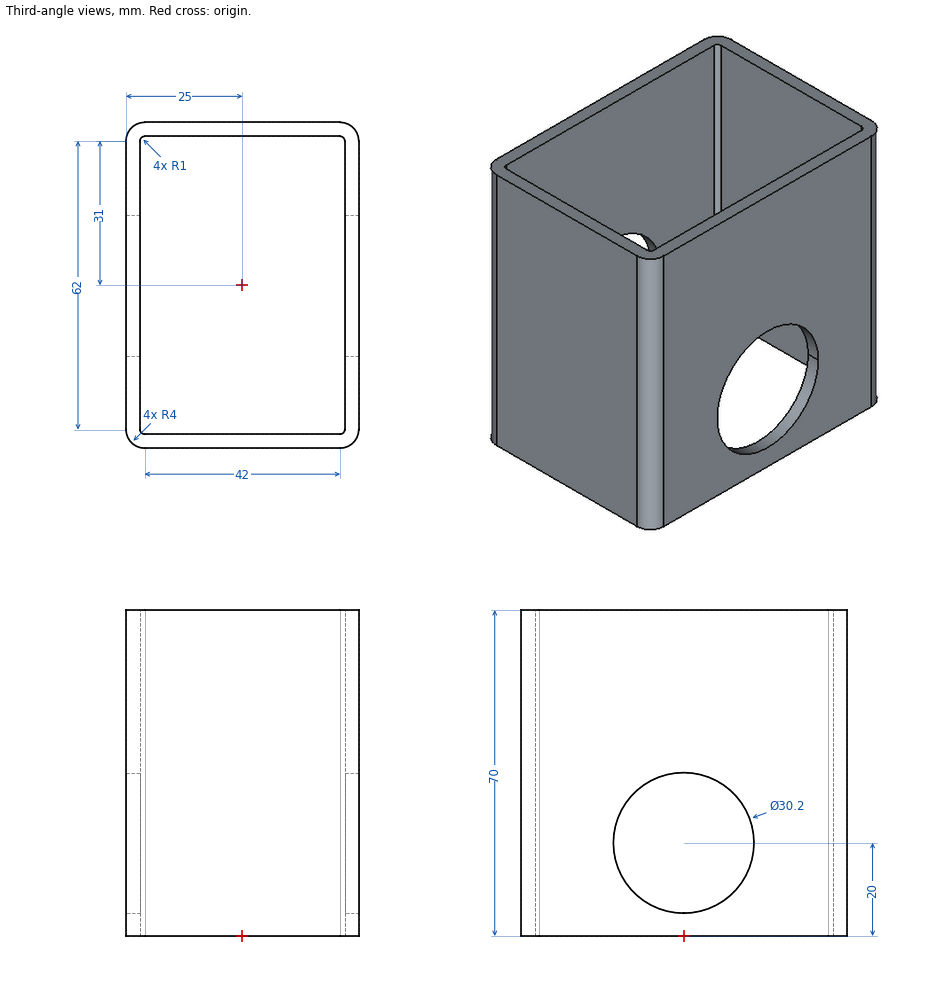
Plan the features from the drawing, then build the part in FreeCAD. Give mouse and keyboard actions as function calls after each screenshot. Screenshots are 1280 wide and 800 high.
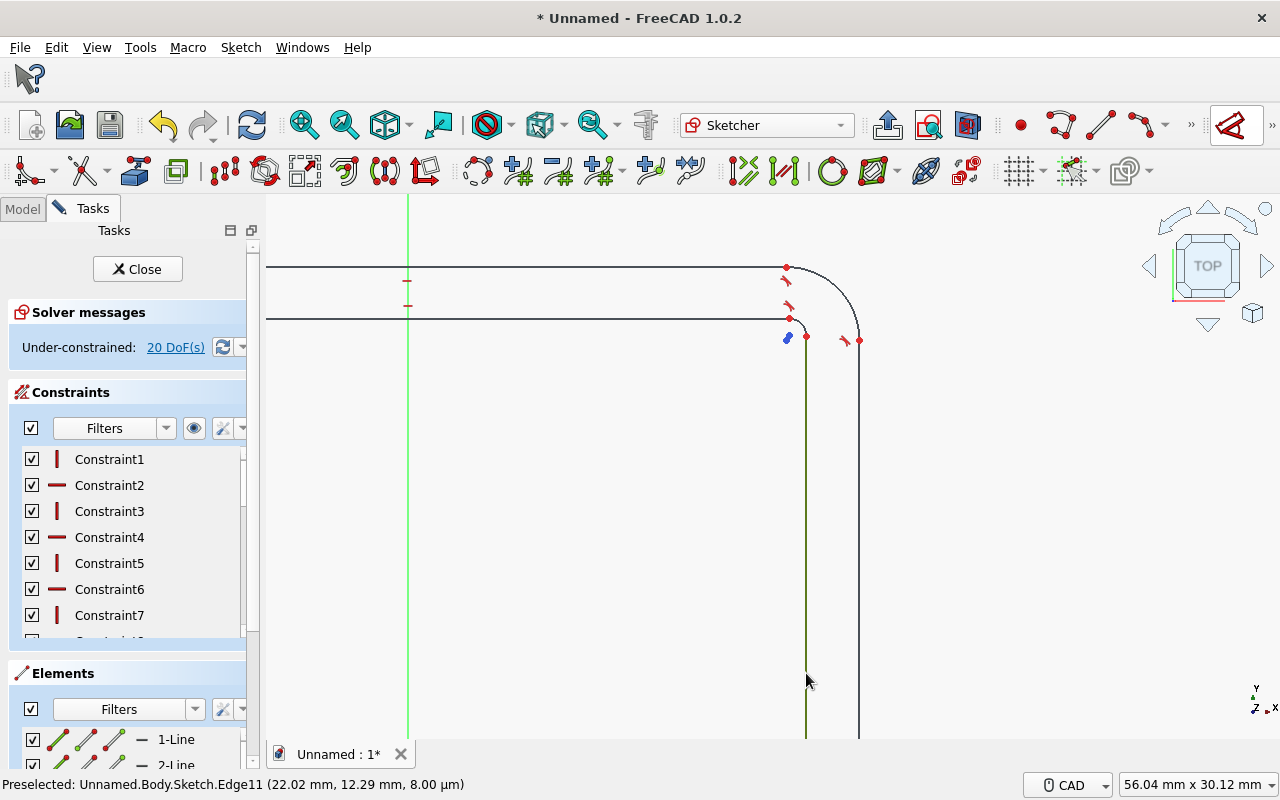
click(802, 324)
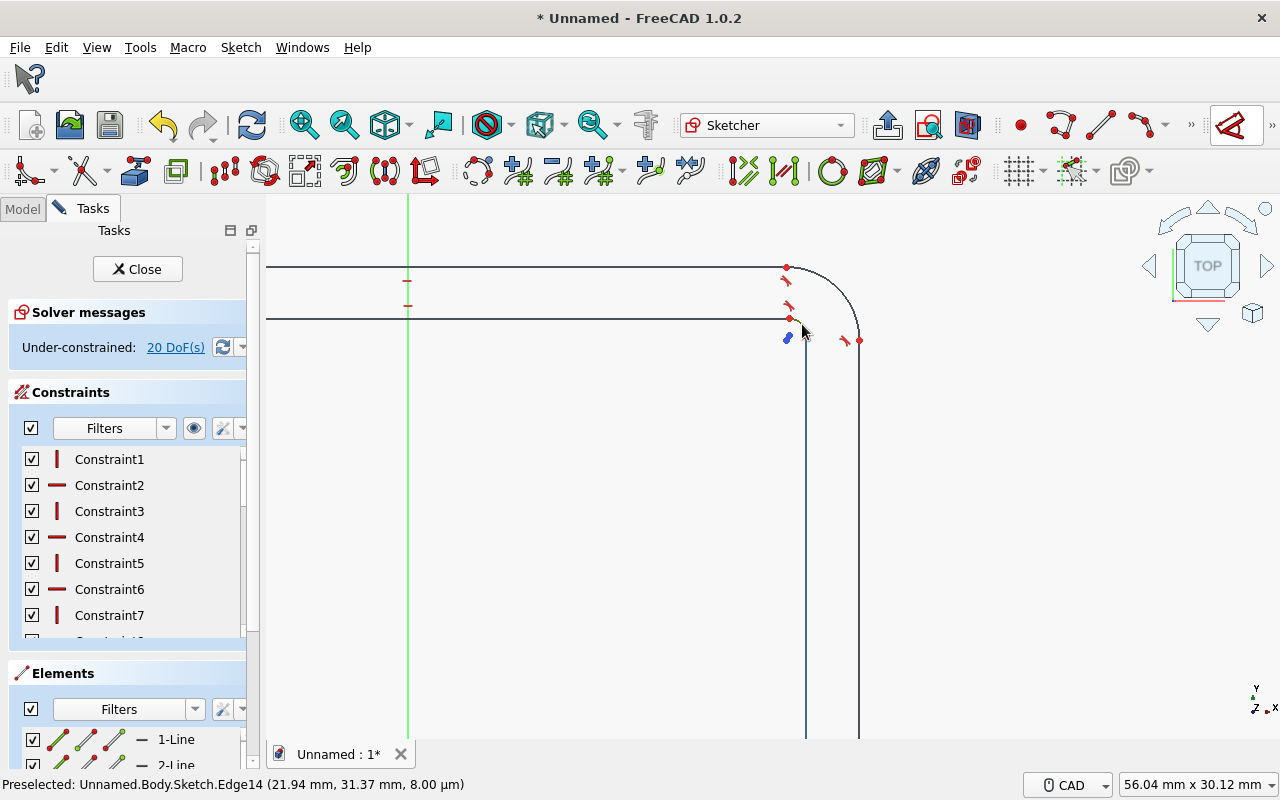
key(t)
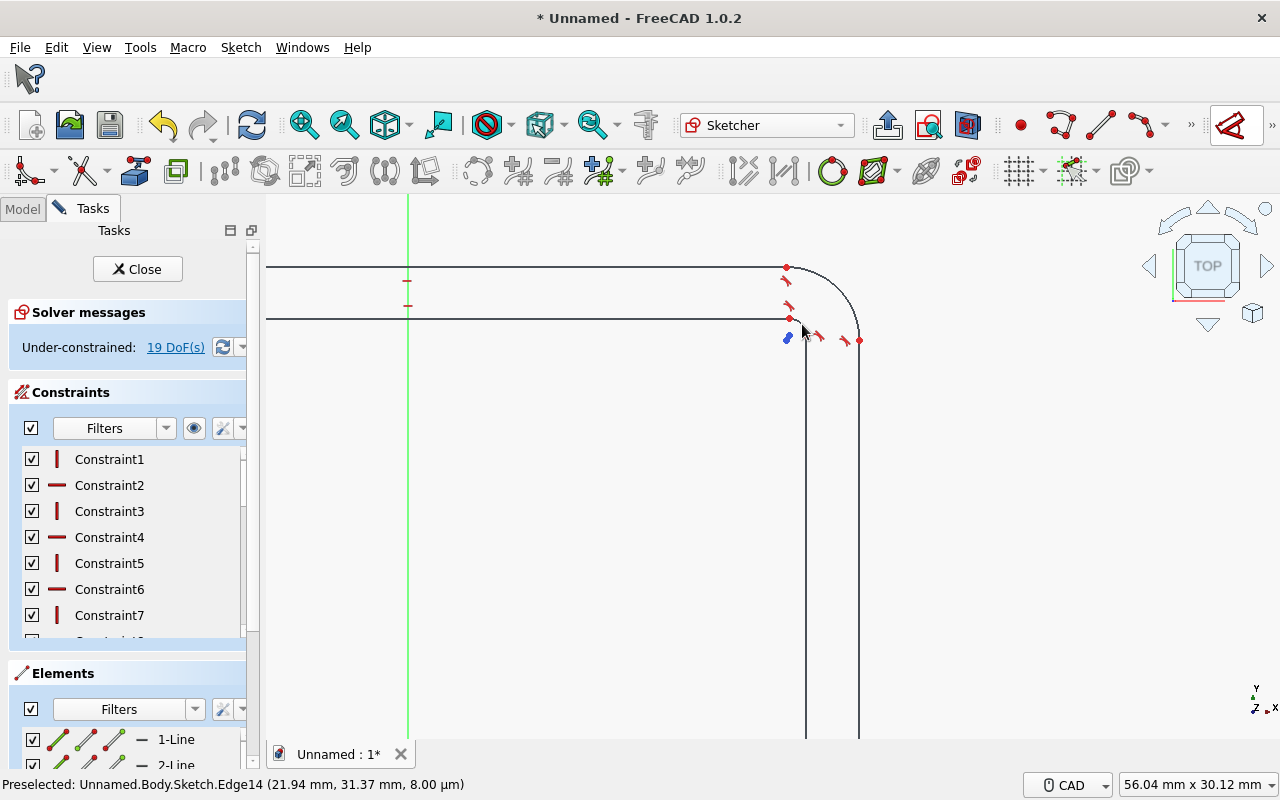
click(806, 672)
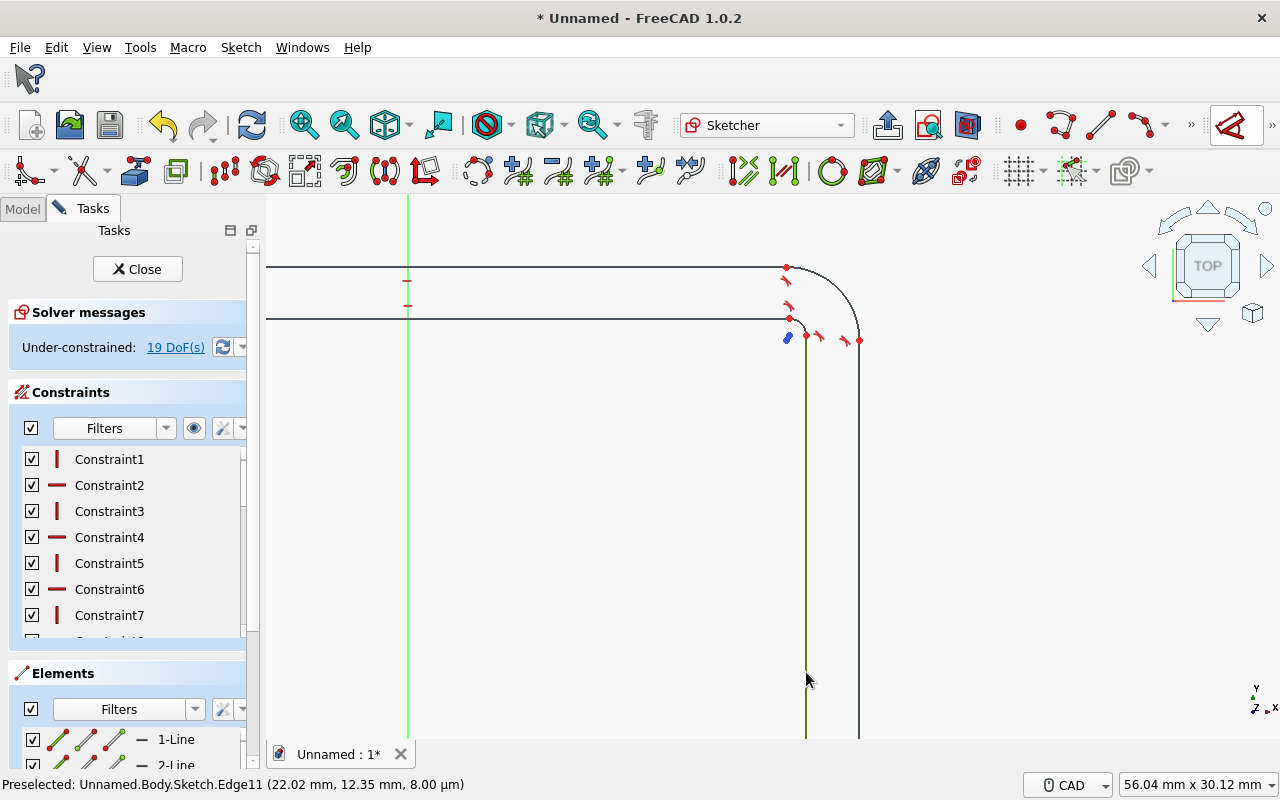
scroll(802, 326, down, 7)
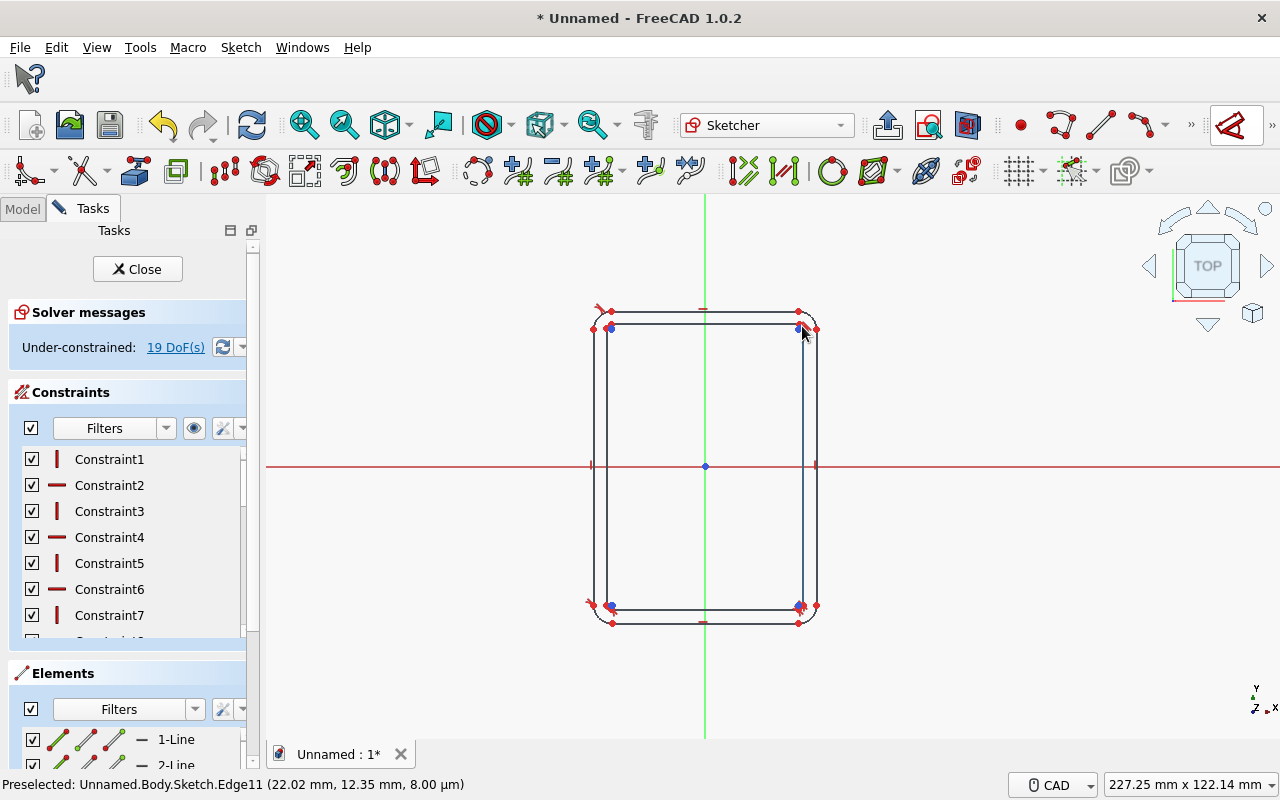
scroll(802, 609, up, 7)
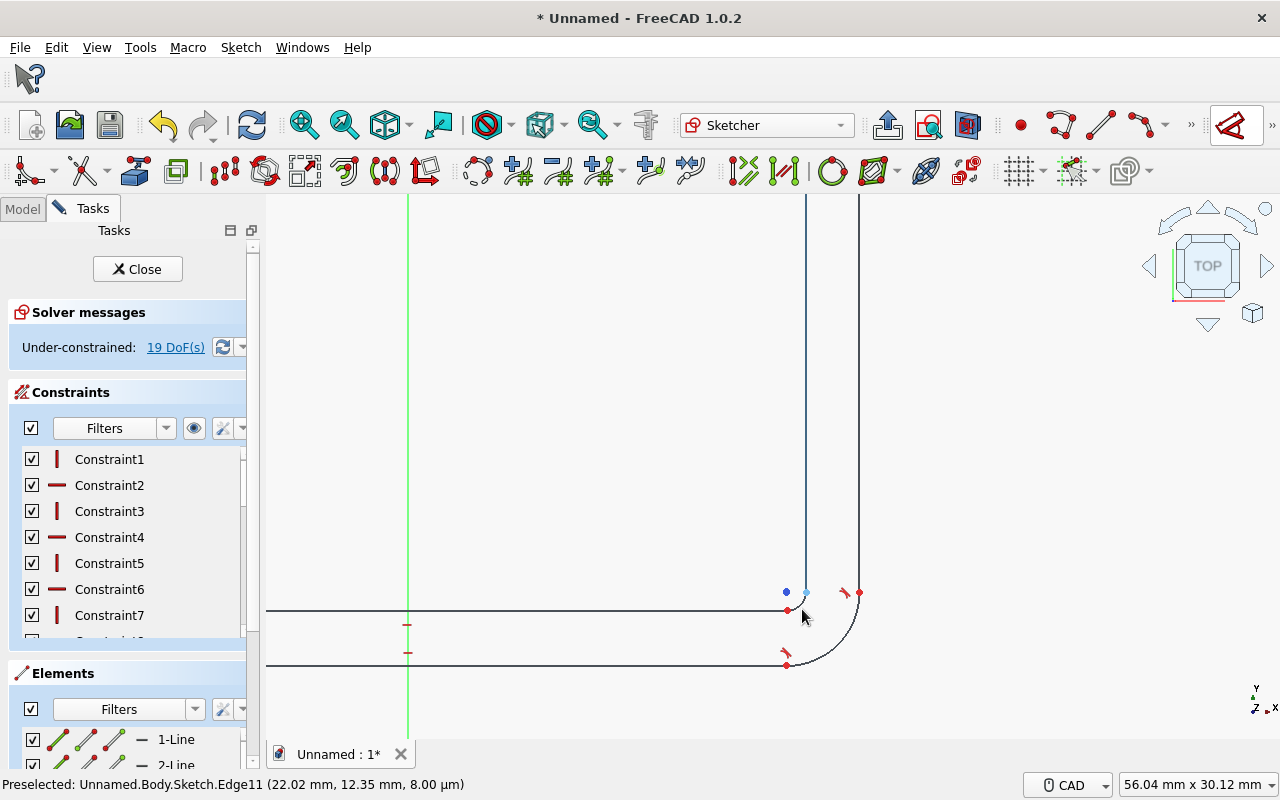
click(801, 605)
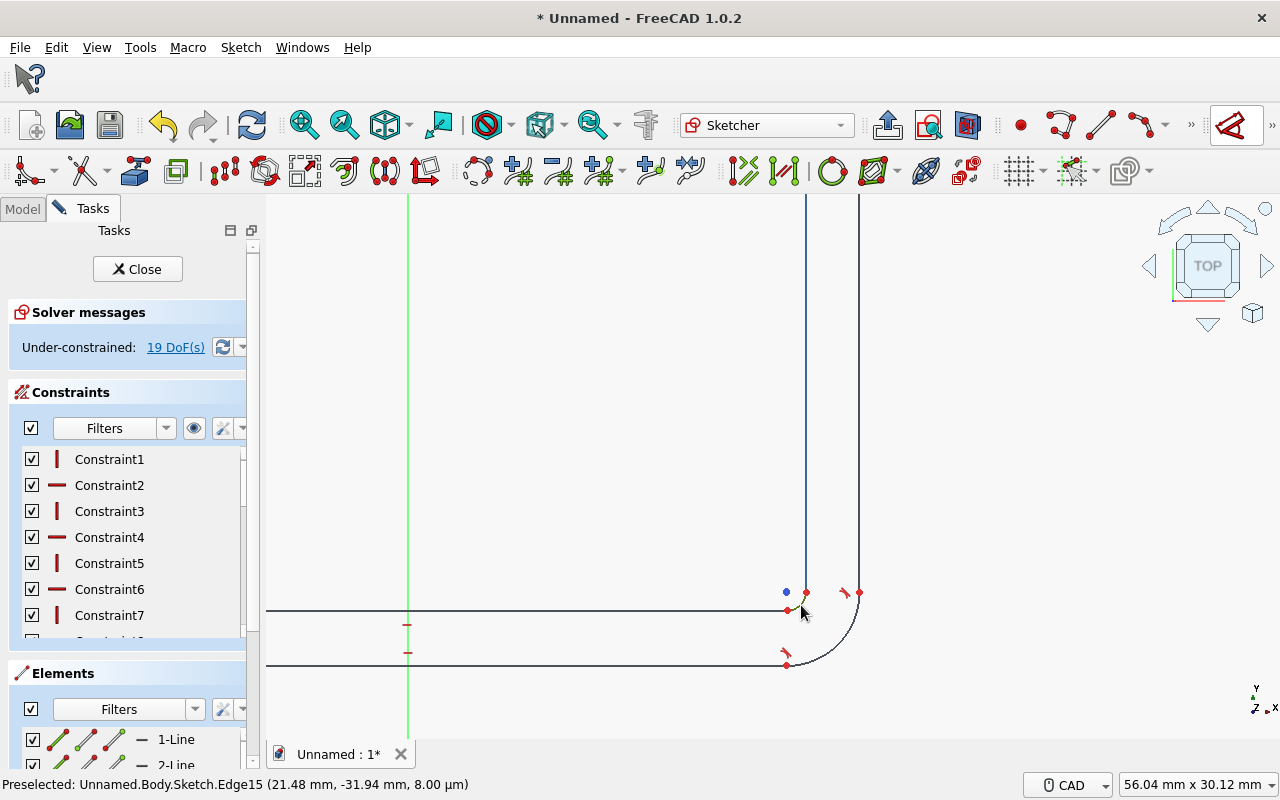
key(t)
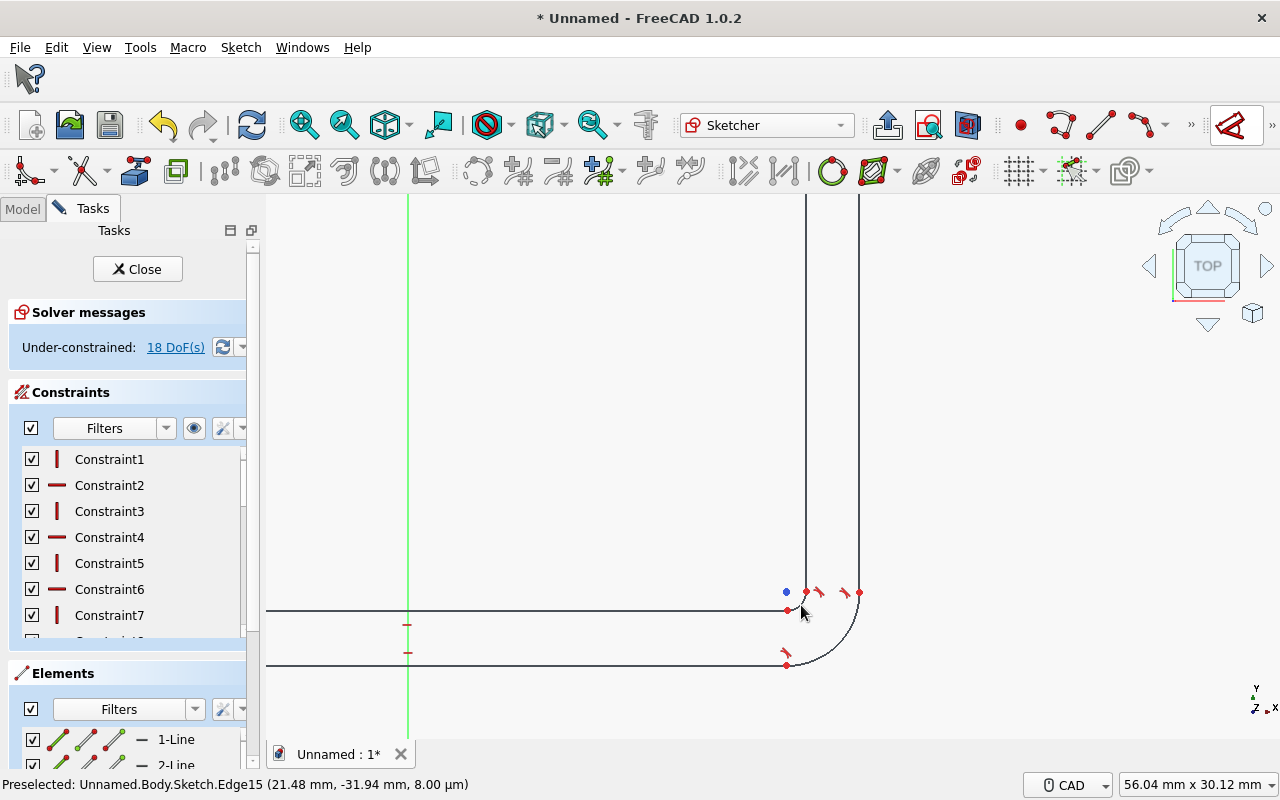
click(560, 611)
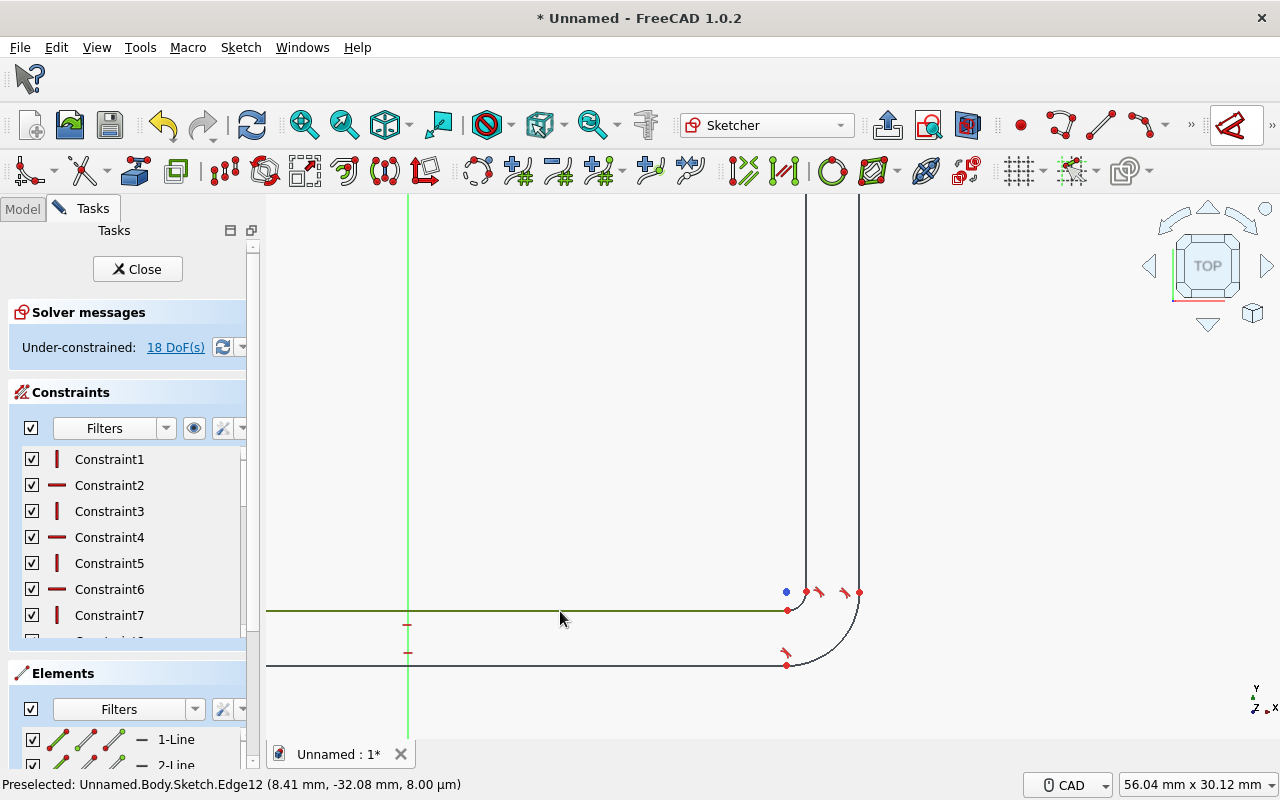
click(801, 605)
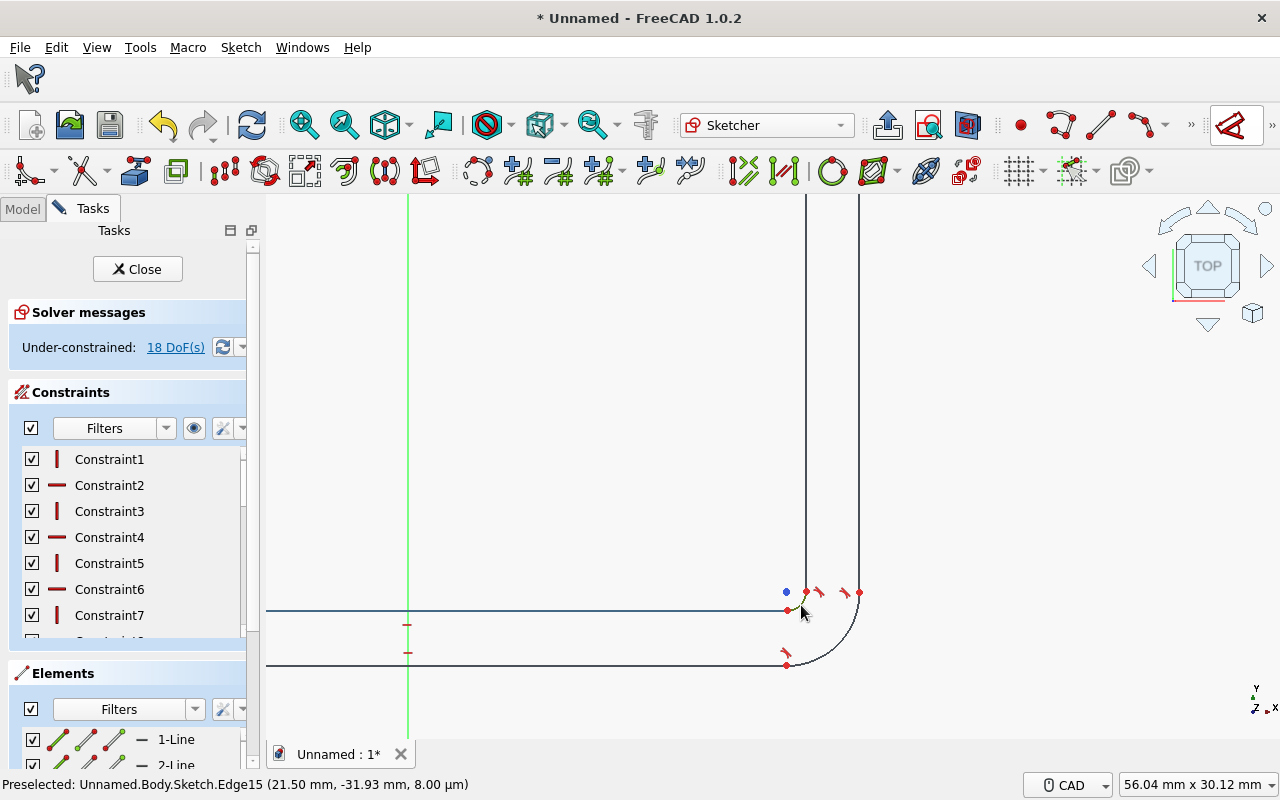
key(t)